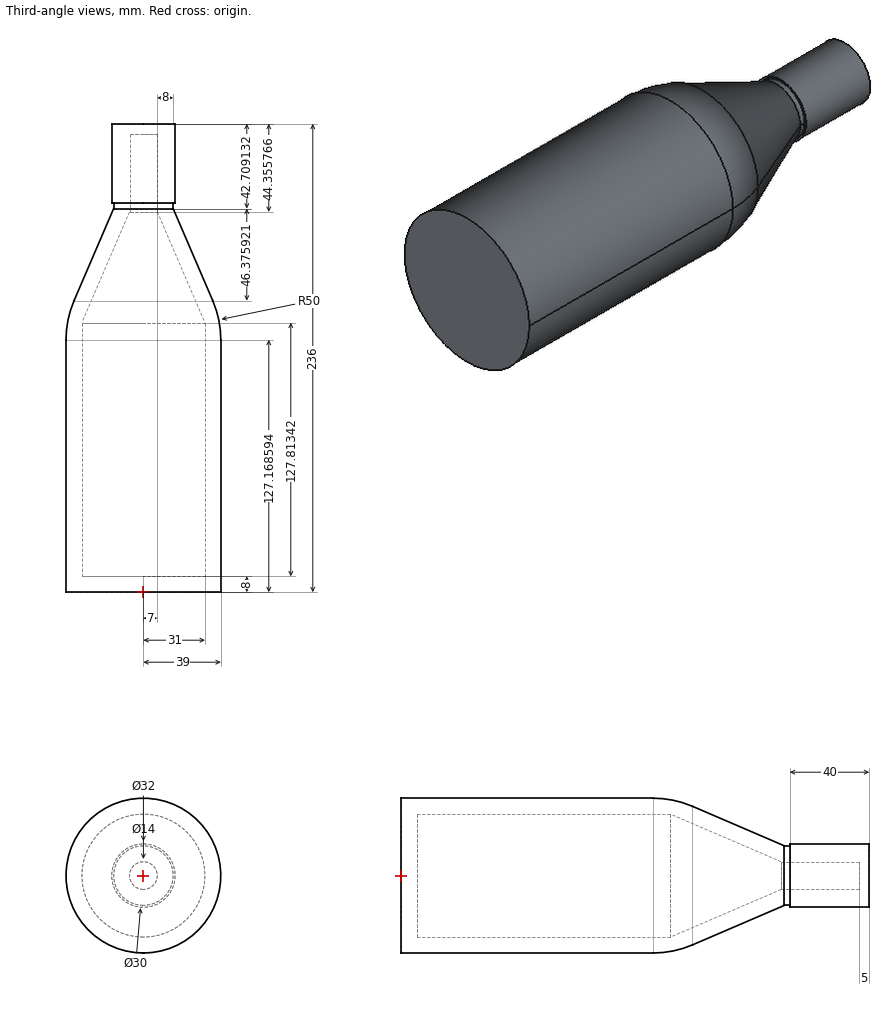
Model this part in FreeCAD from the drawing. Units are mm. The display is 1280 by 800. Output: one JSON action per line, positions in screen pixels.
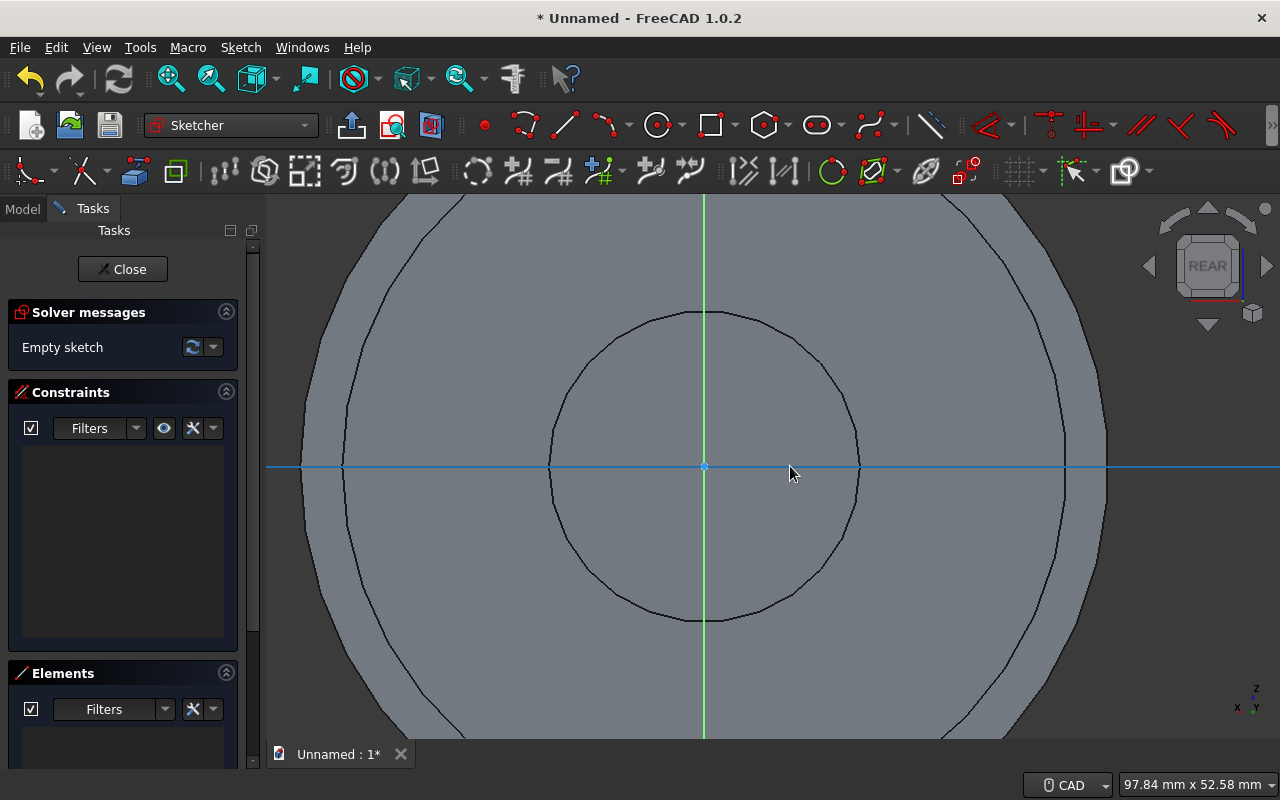
{"action": "key", "text": "g c"}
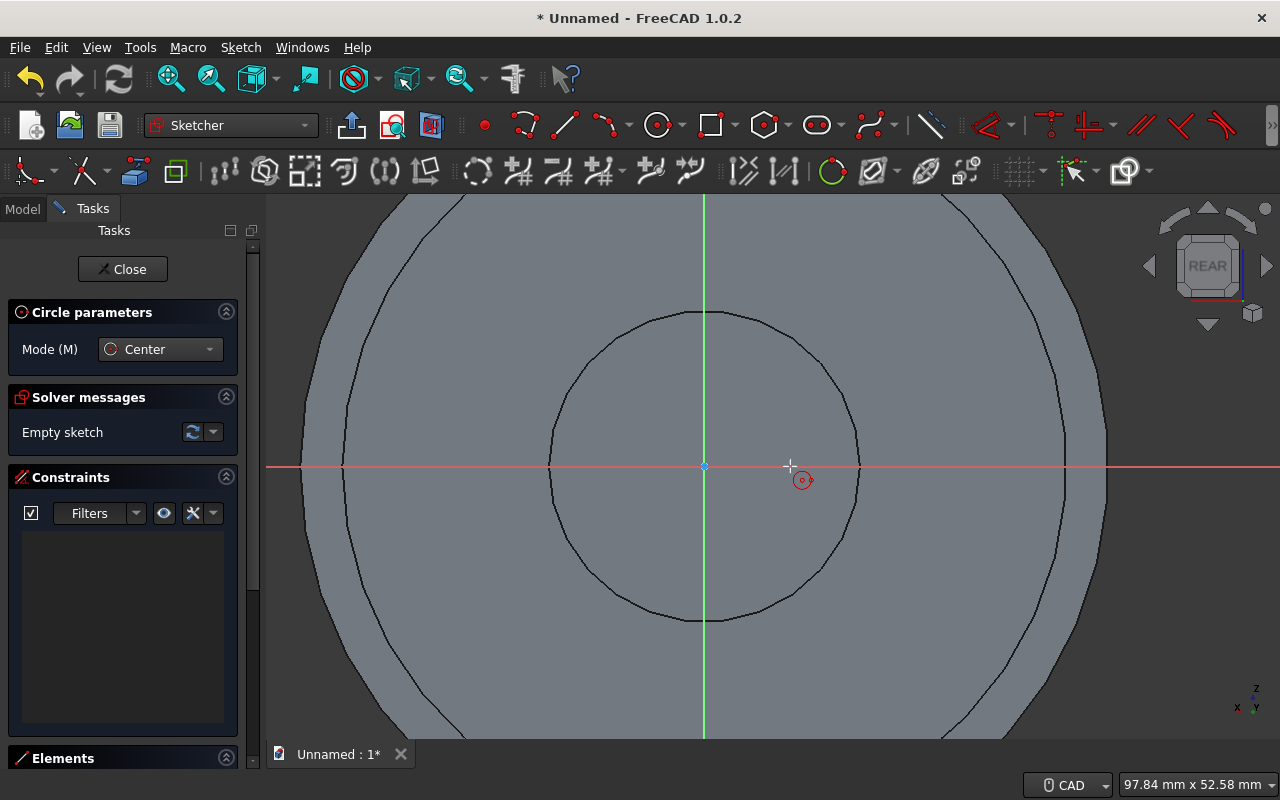
{"action": "left_click", "coordinate": [704, 466]}
{"action": "mouse_move", "coordinate": [822, 349]}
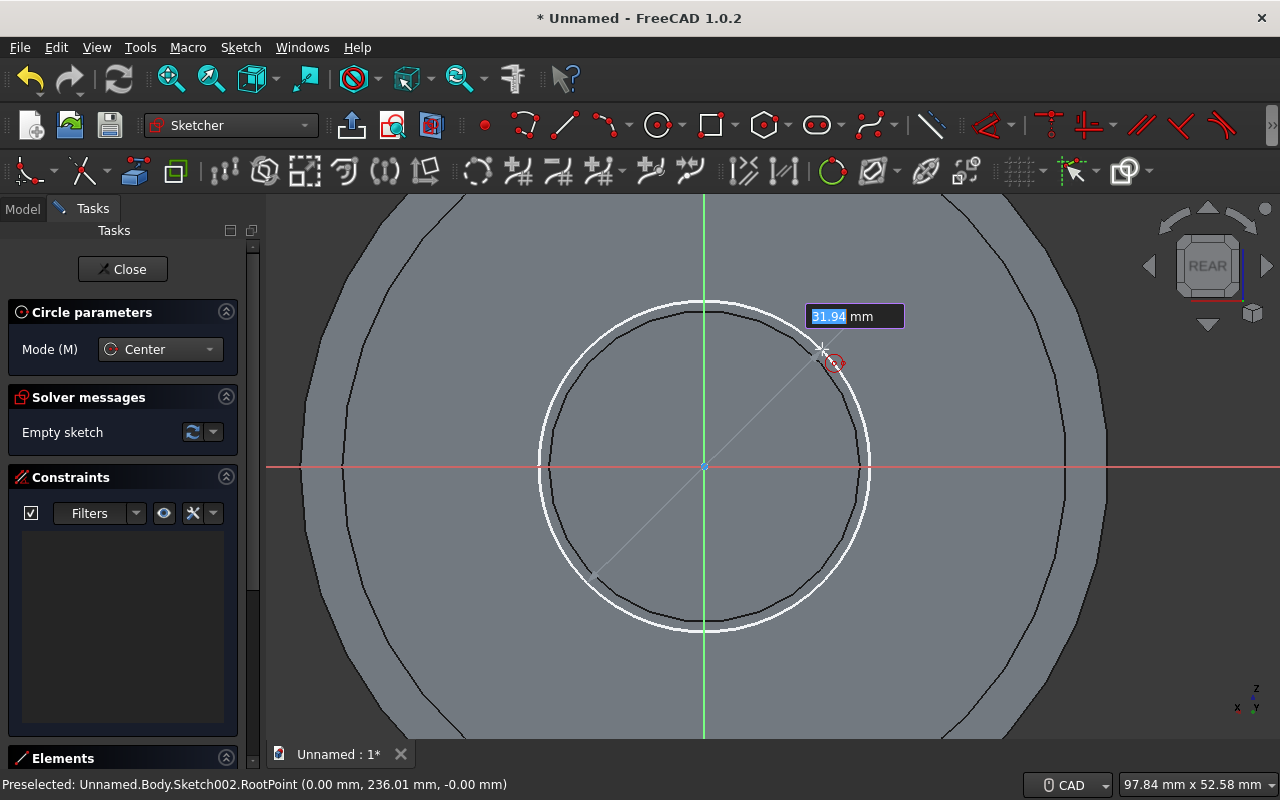
{"action": "type", "text": "32"}
{"action": "key", "text": "Return"}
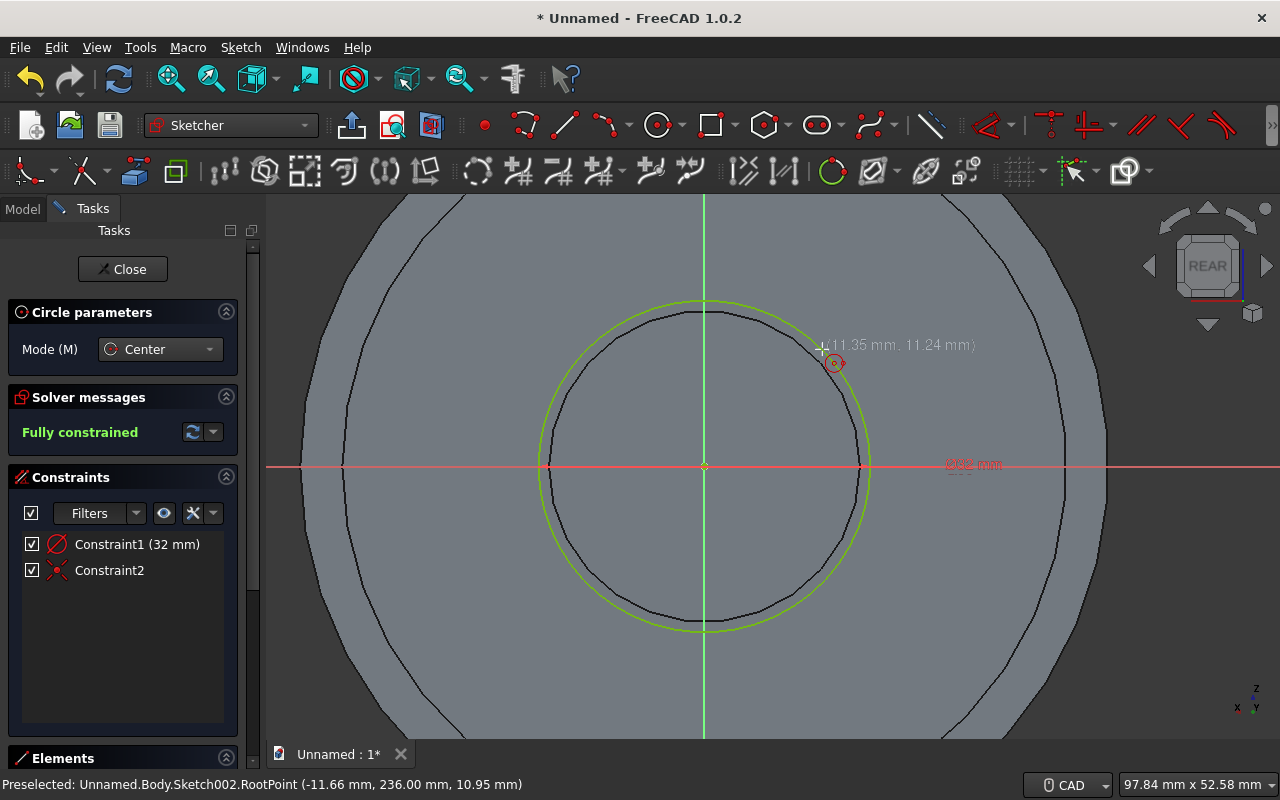
{"action": "left_click", "coordinate": [704, 466]}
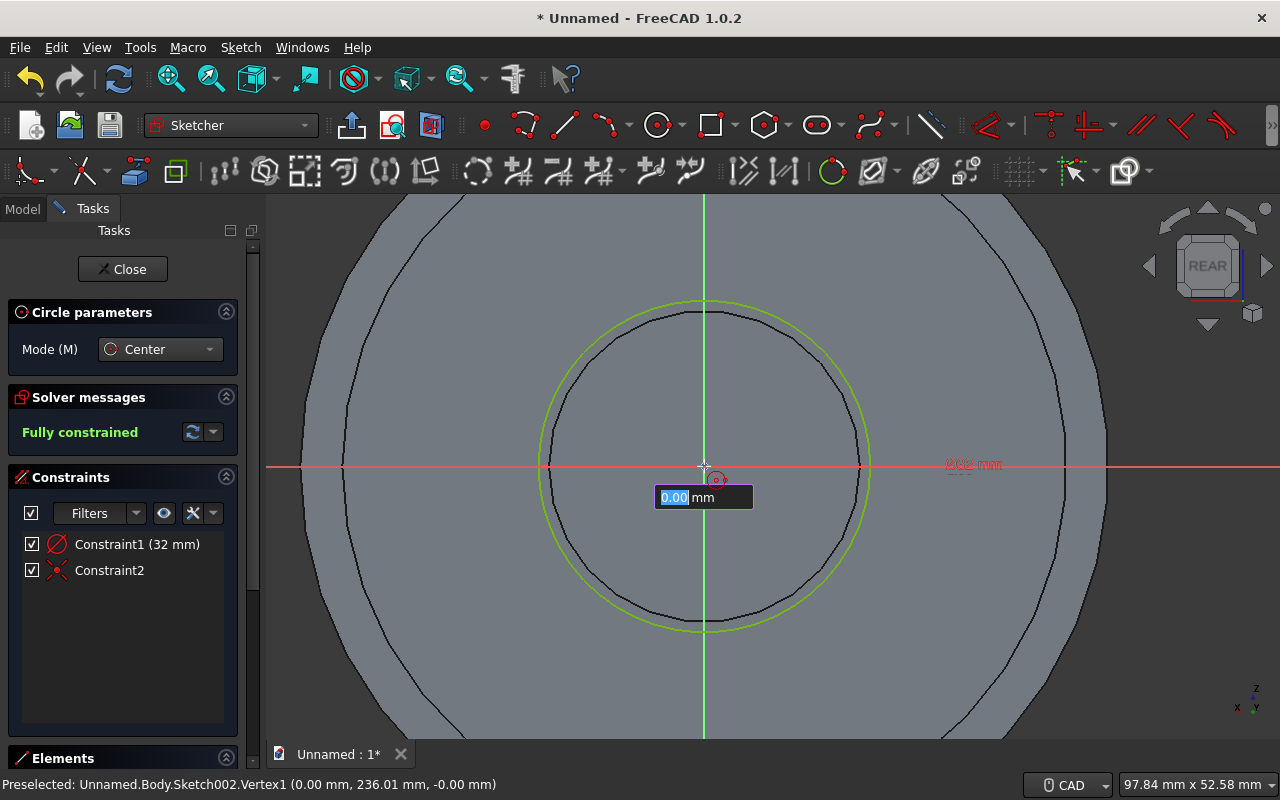
{"action": "scroll", "coordinate": [814, 357], "scroll_direction": "up", "scroll_amount": 3}
{"action": "mouse_move", "coordinate": [814, 356]}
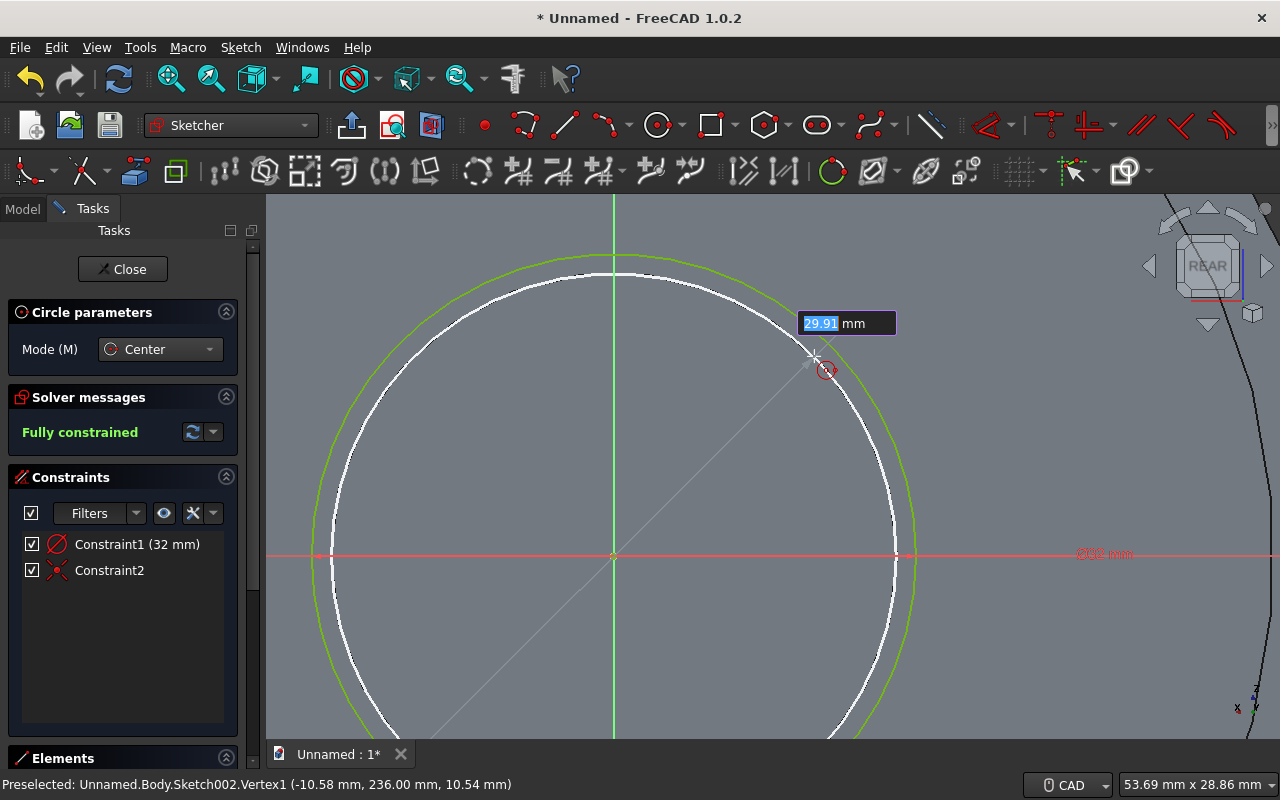
{"action": "type", "text": "30"}
{"action": "key", "text": "Return"}
{"action": "key", "text": "Escape"}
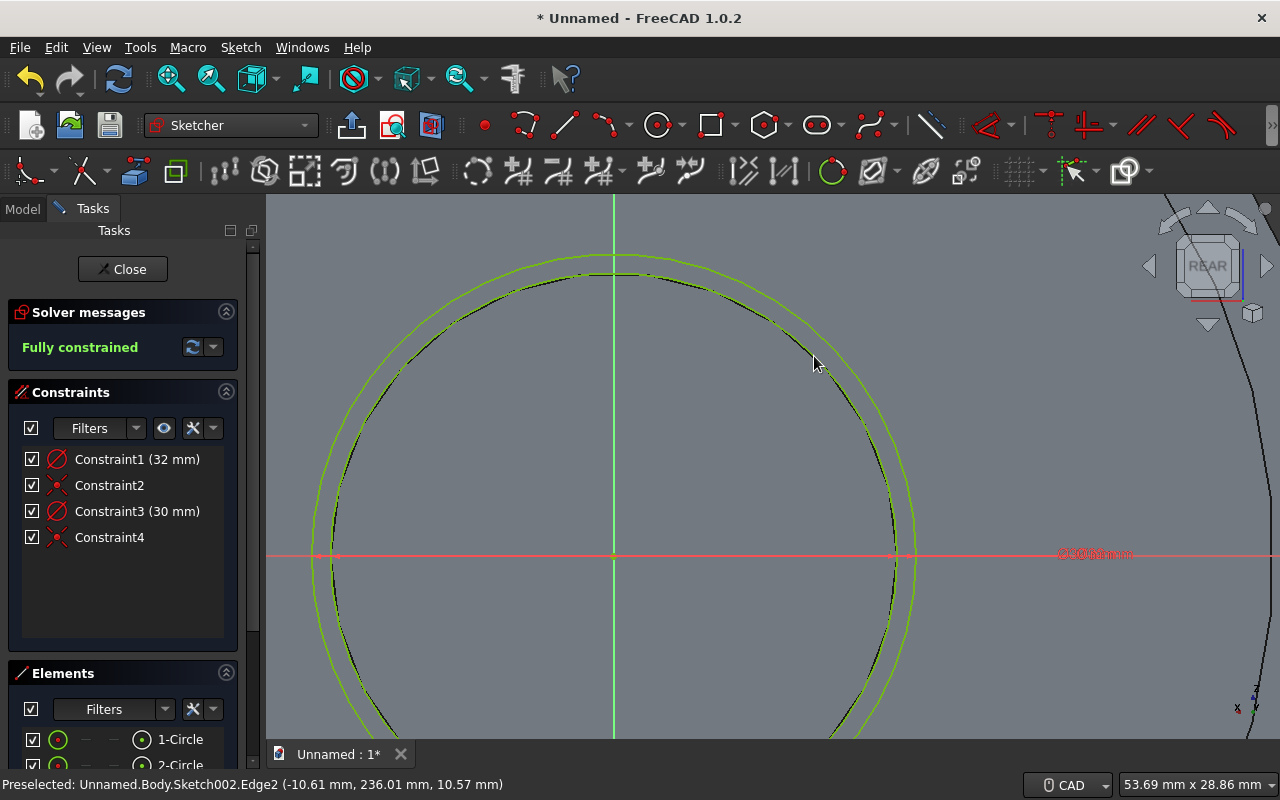
{"action": "left_click", "coordinate": [123, 269]}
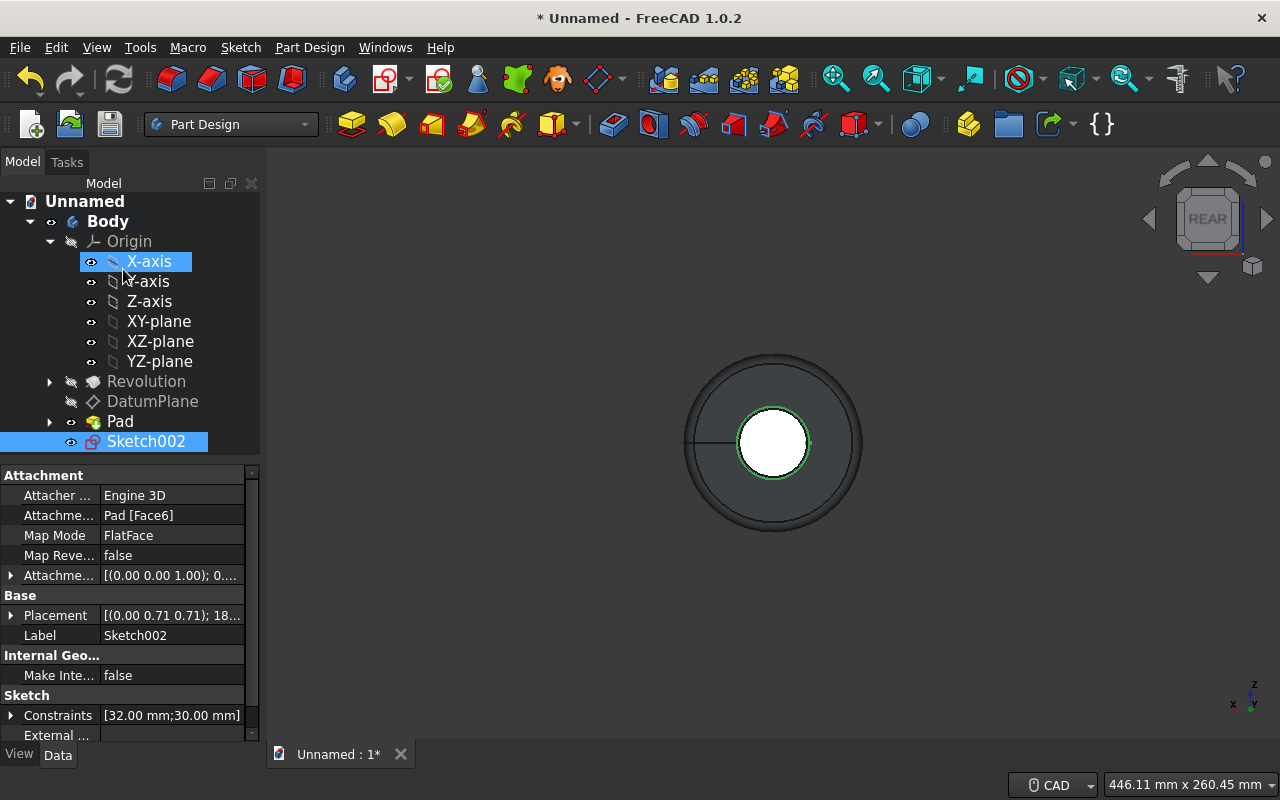
{"action": "left_click", "coordinate": [352, 124]}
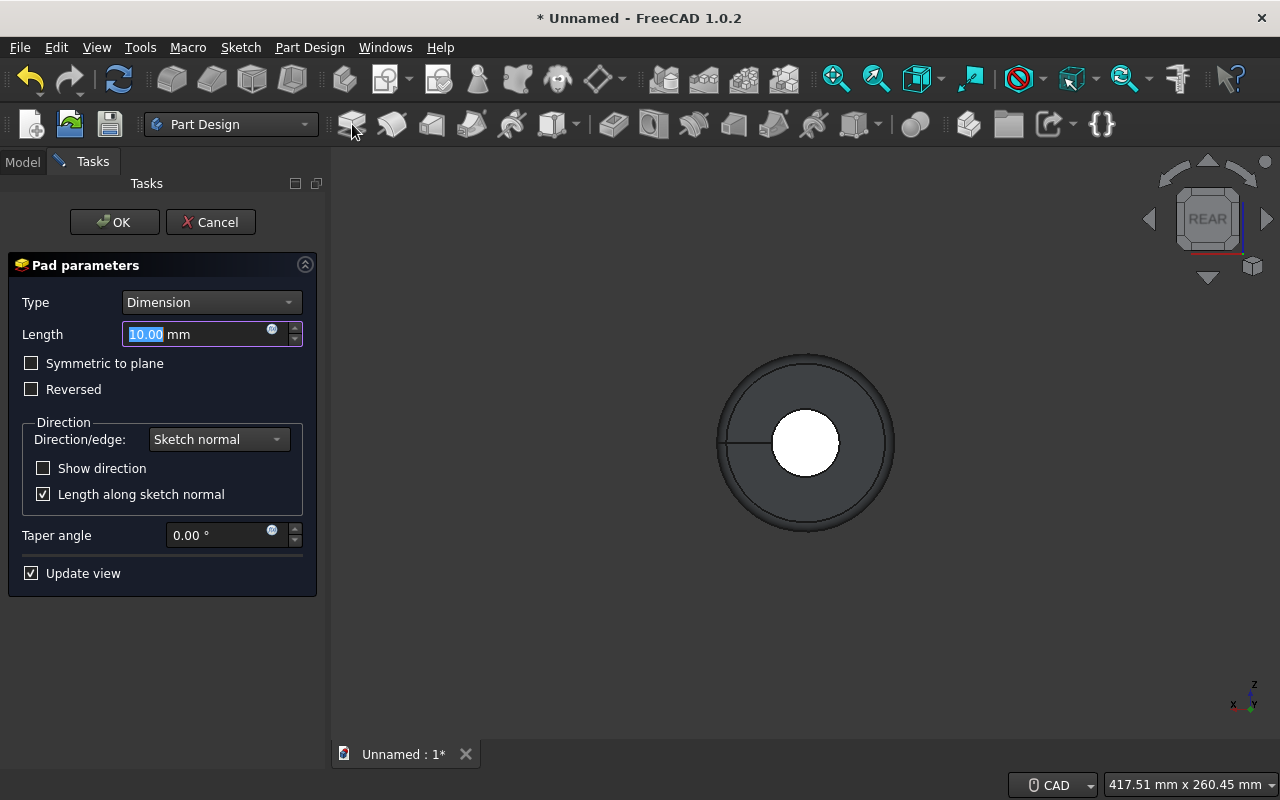
{"action": "type", "text": "40"}
{"action": "key", "text": "Tab"}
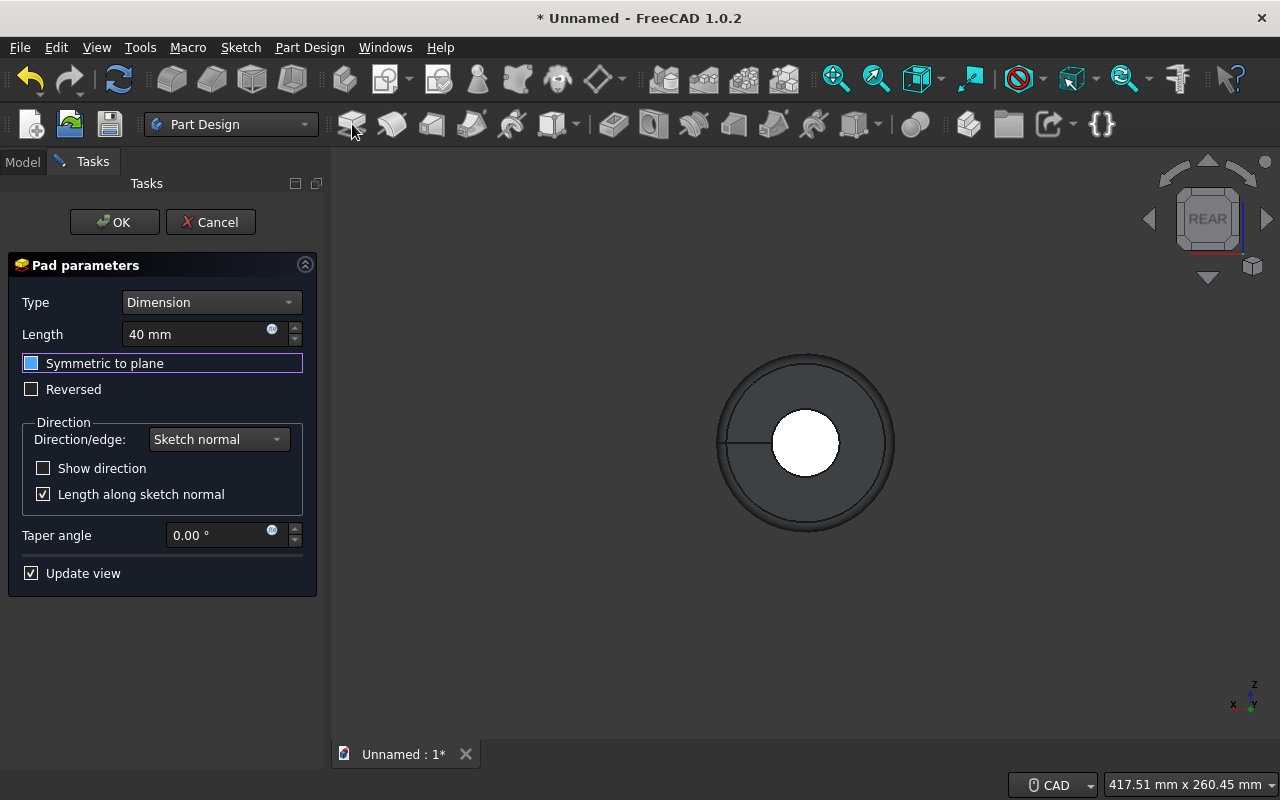
{"action": "left_click", "coordinate": [30, 389]}